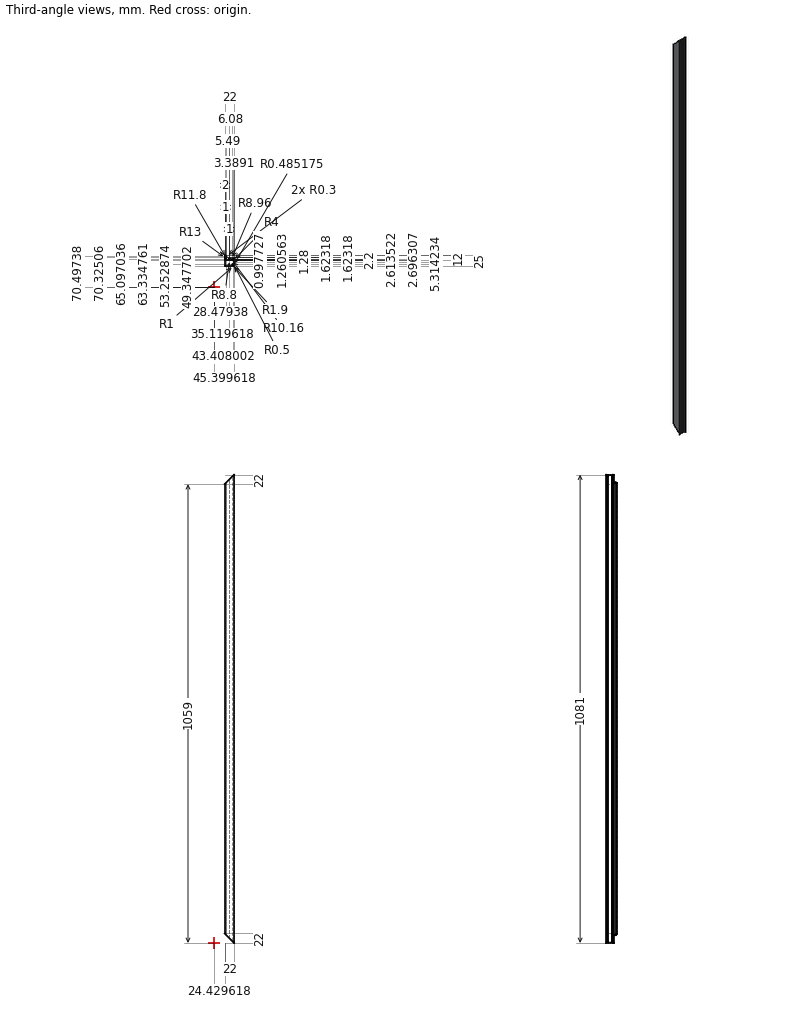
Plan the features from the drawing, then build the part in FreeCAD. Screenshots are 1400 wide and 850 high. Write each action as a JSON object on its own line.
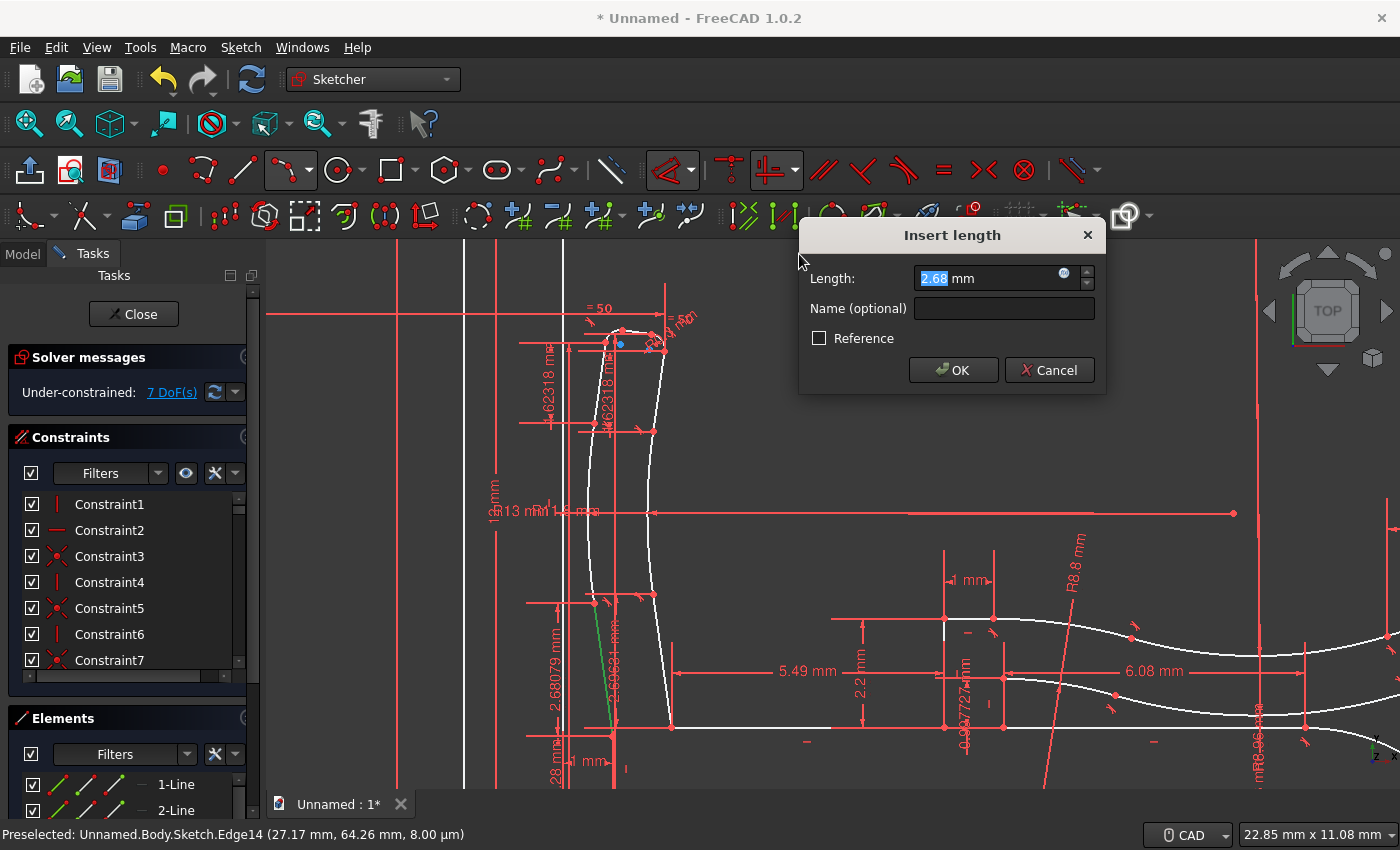
{"action": "type", "text": "2.613522"}
{"action": "key", "text": "Return"}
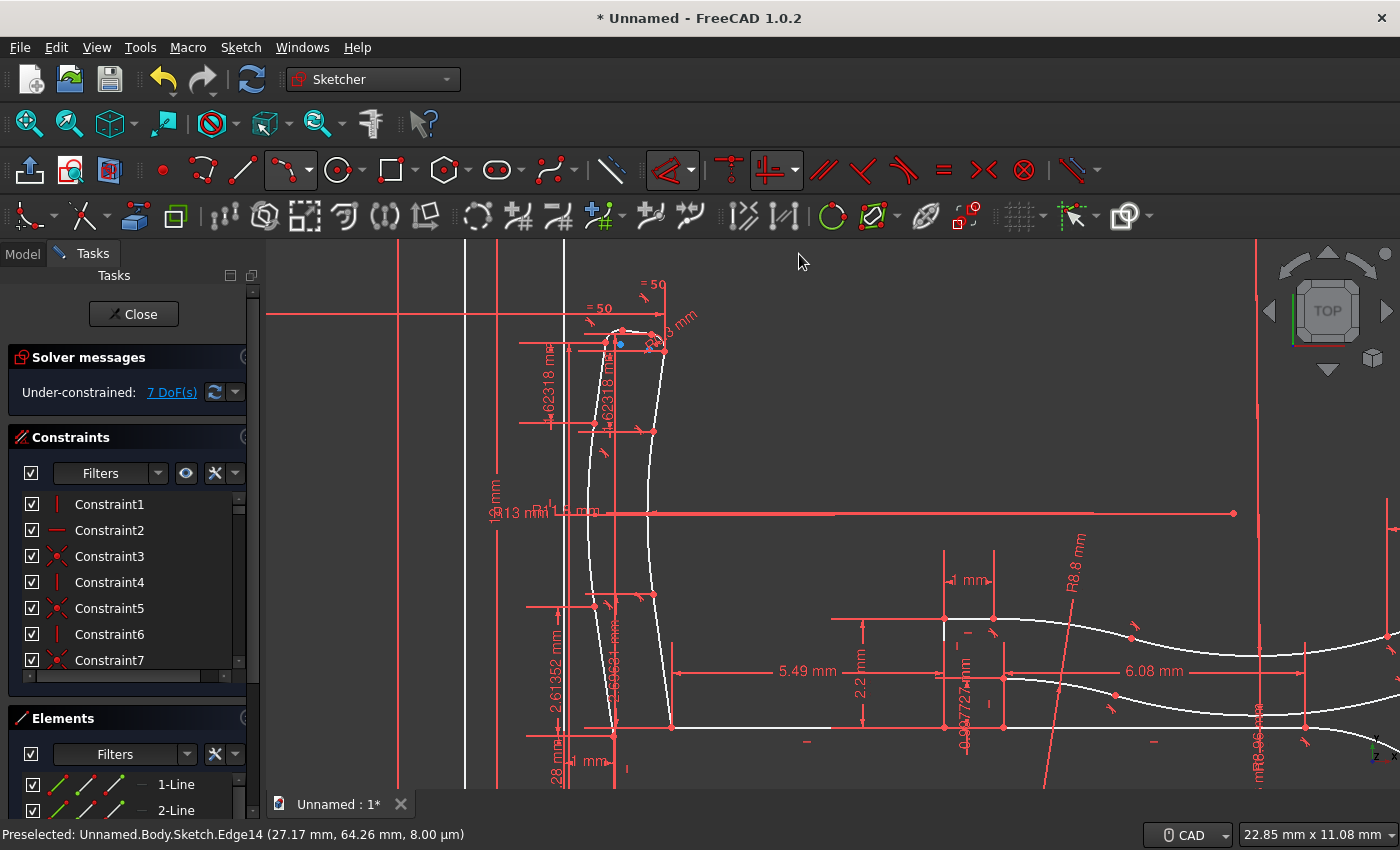
{"action": "scroll", "coordinate": [659, 382], "scroll_direction": "down", "scroll_amount": 6}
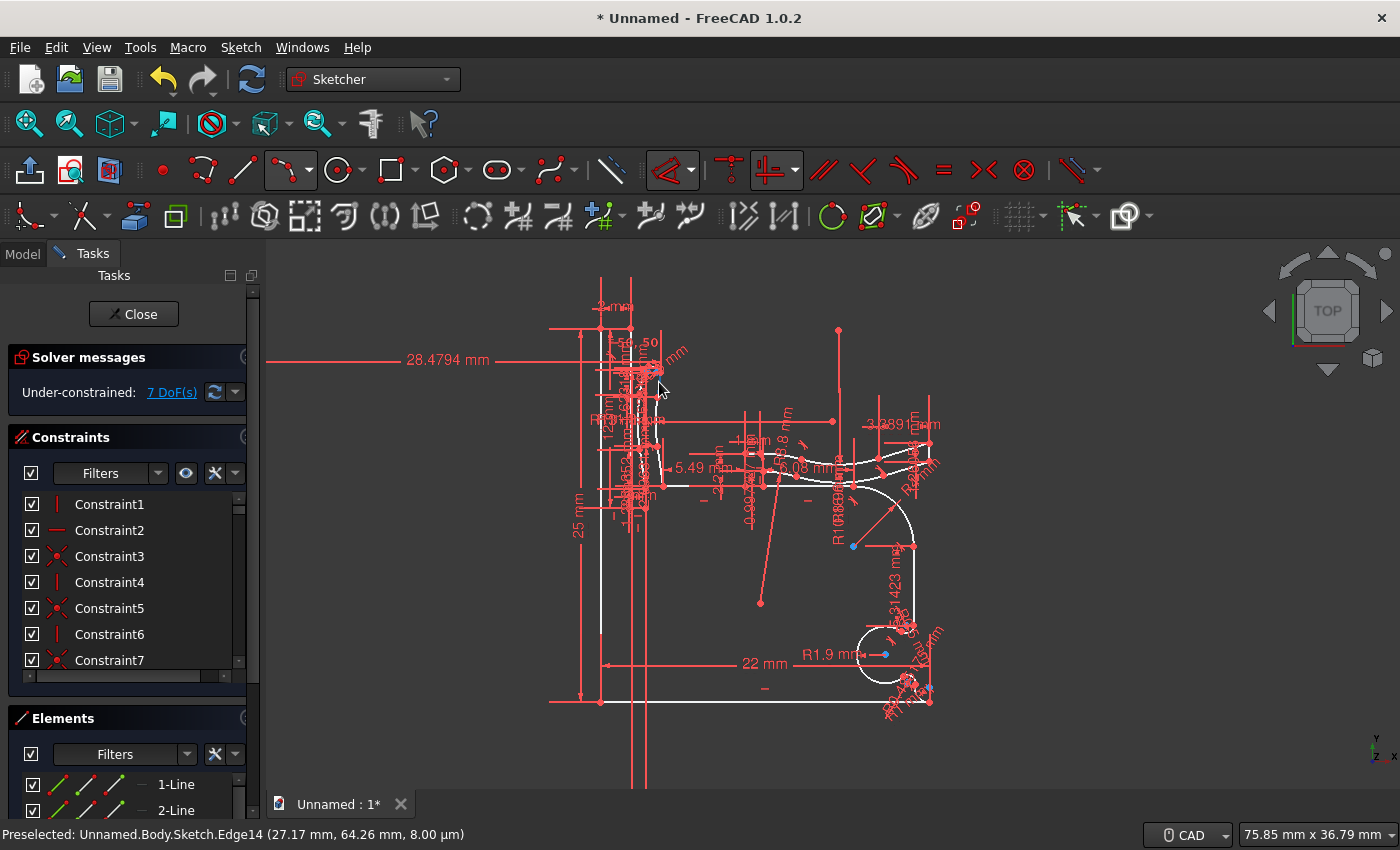
{"action": "scroll", "coordinate": [914, 626], "scroll_direction": "up", "scroll_amount": 3}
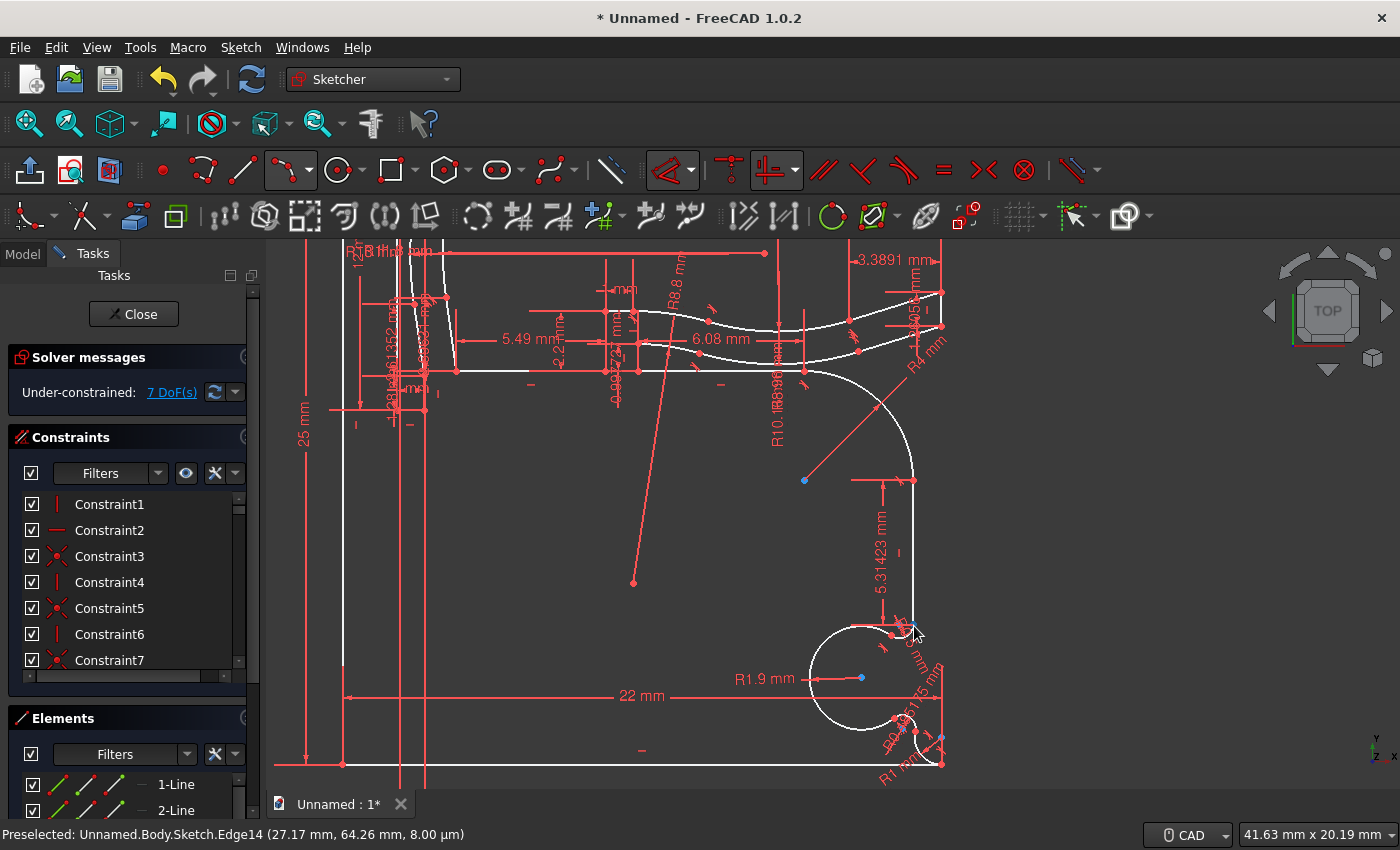
{"action": "left_click", "coordinate": [913, 625]}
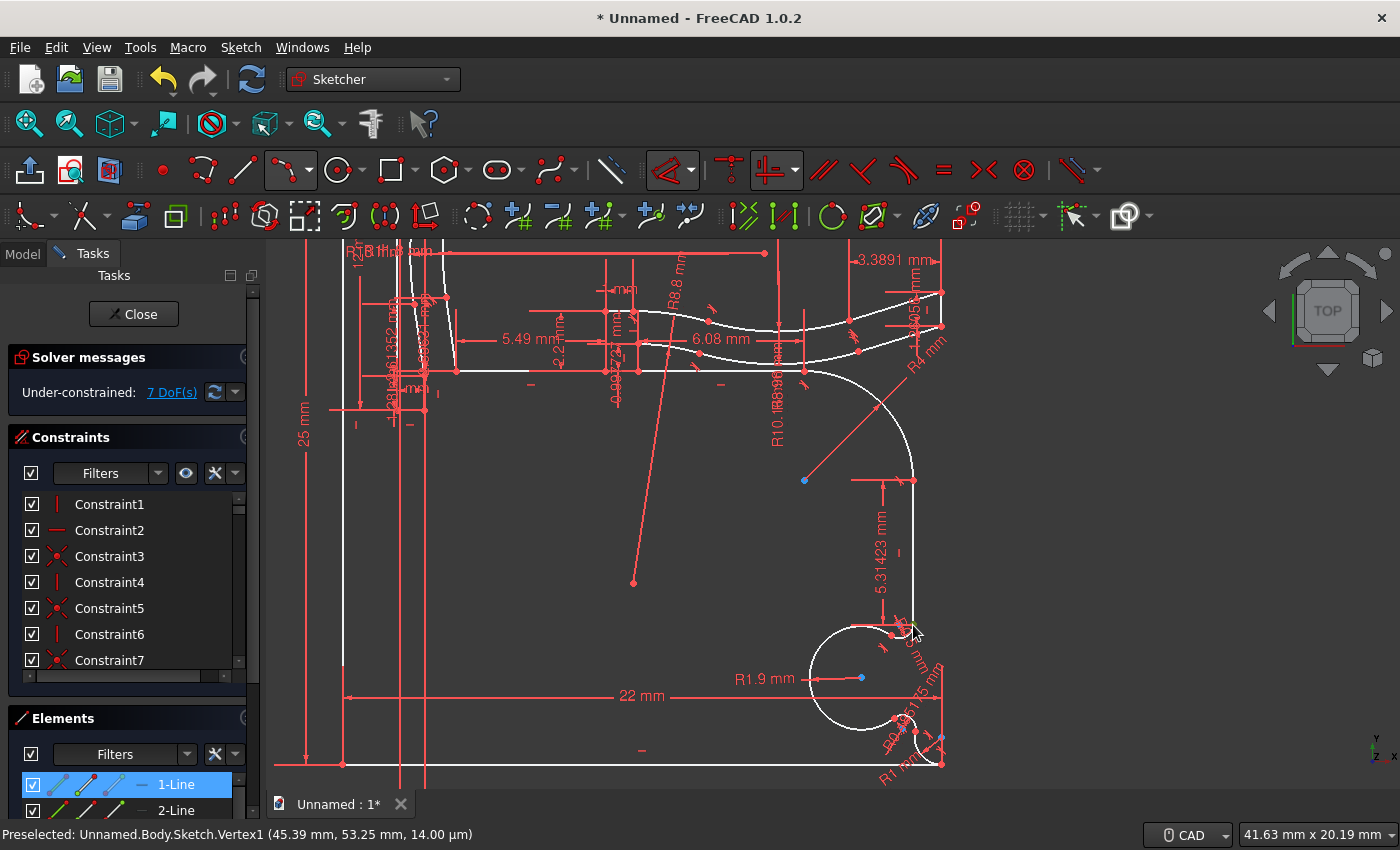
{"action": "left_click", "coordinate": [694, 170]}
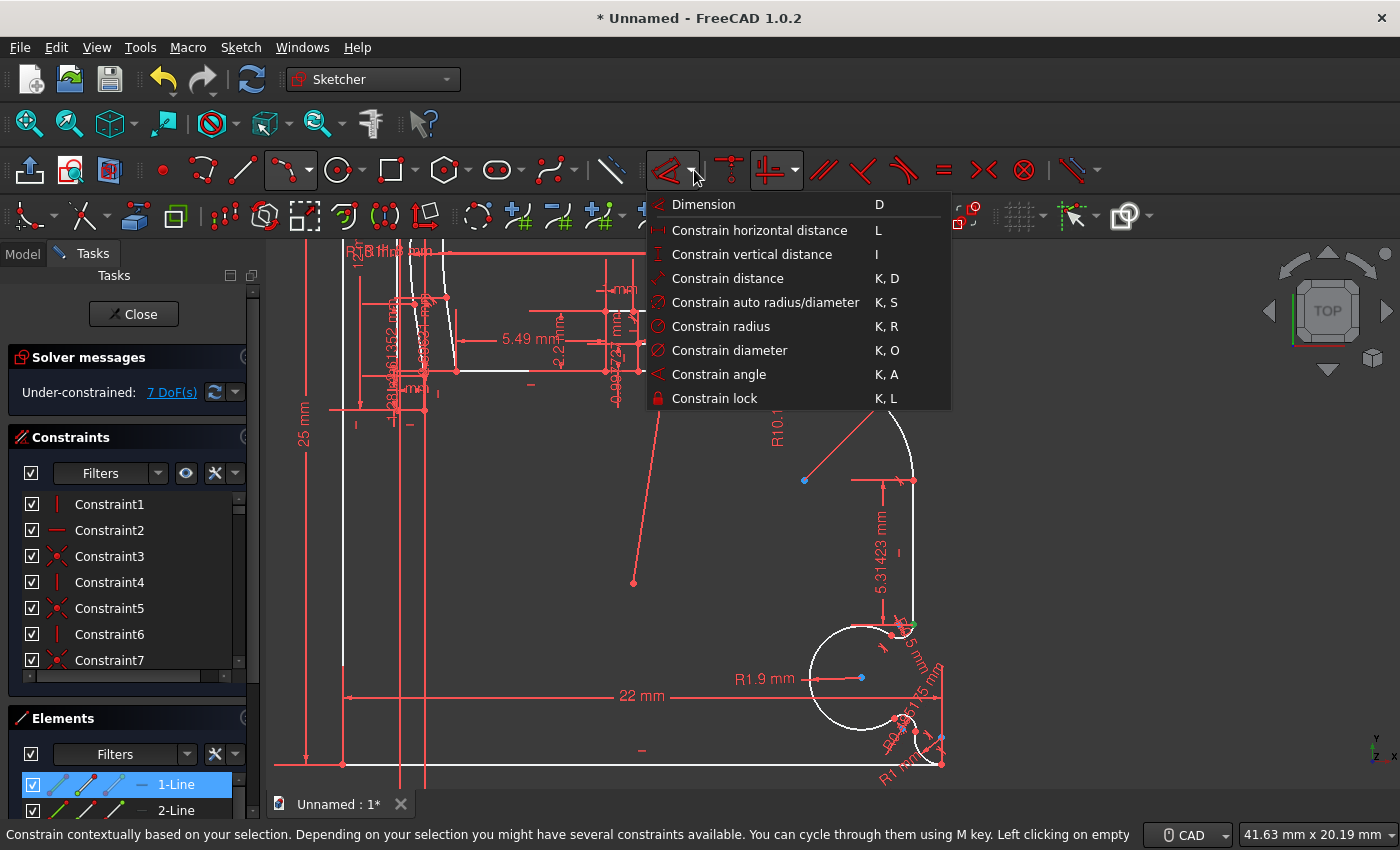
{"action": "left_click", "coordinate": [799, 230]}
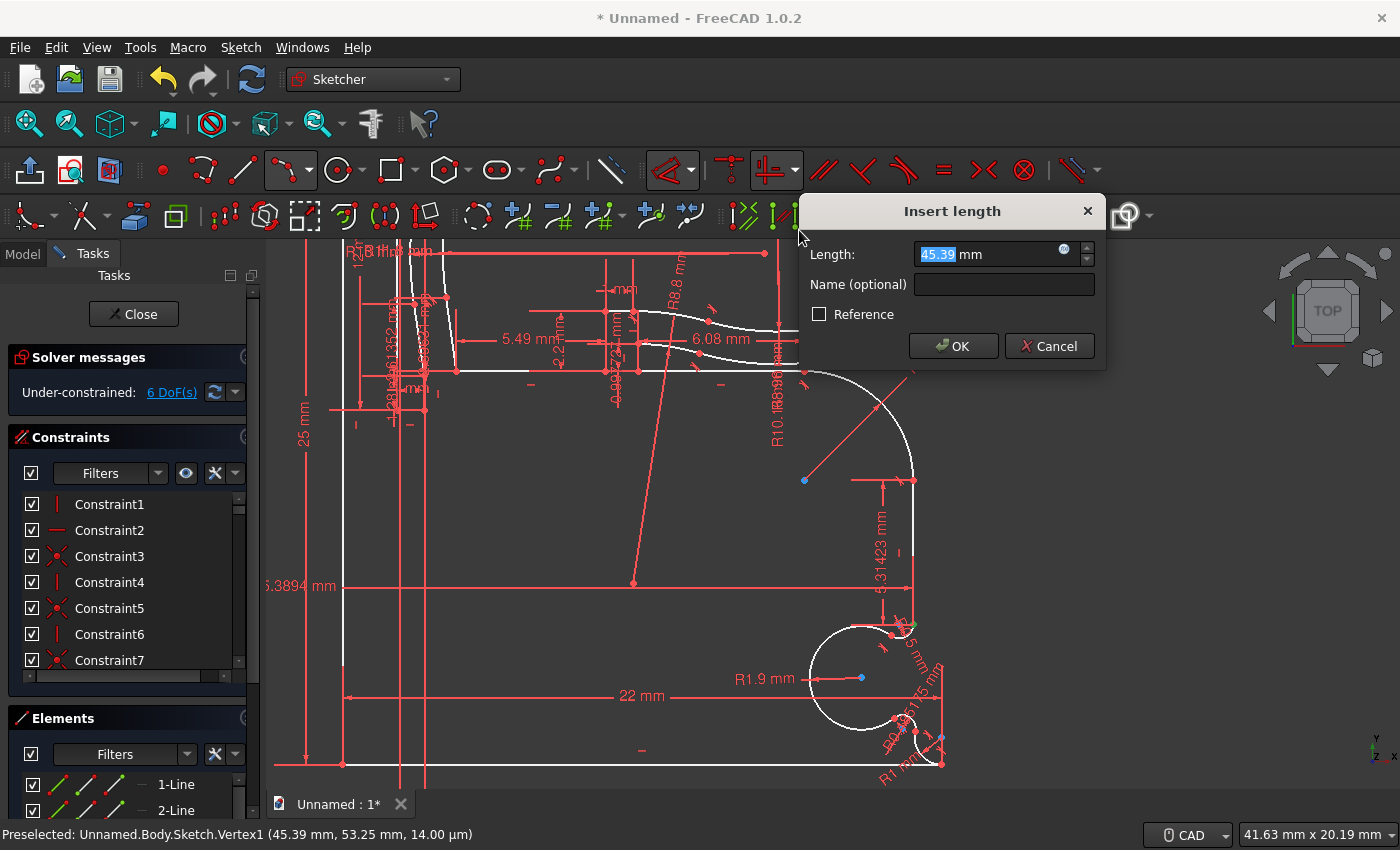
{"action": "type", "text": "45.399618"}
{"action": "key", "text": "Return"}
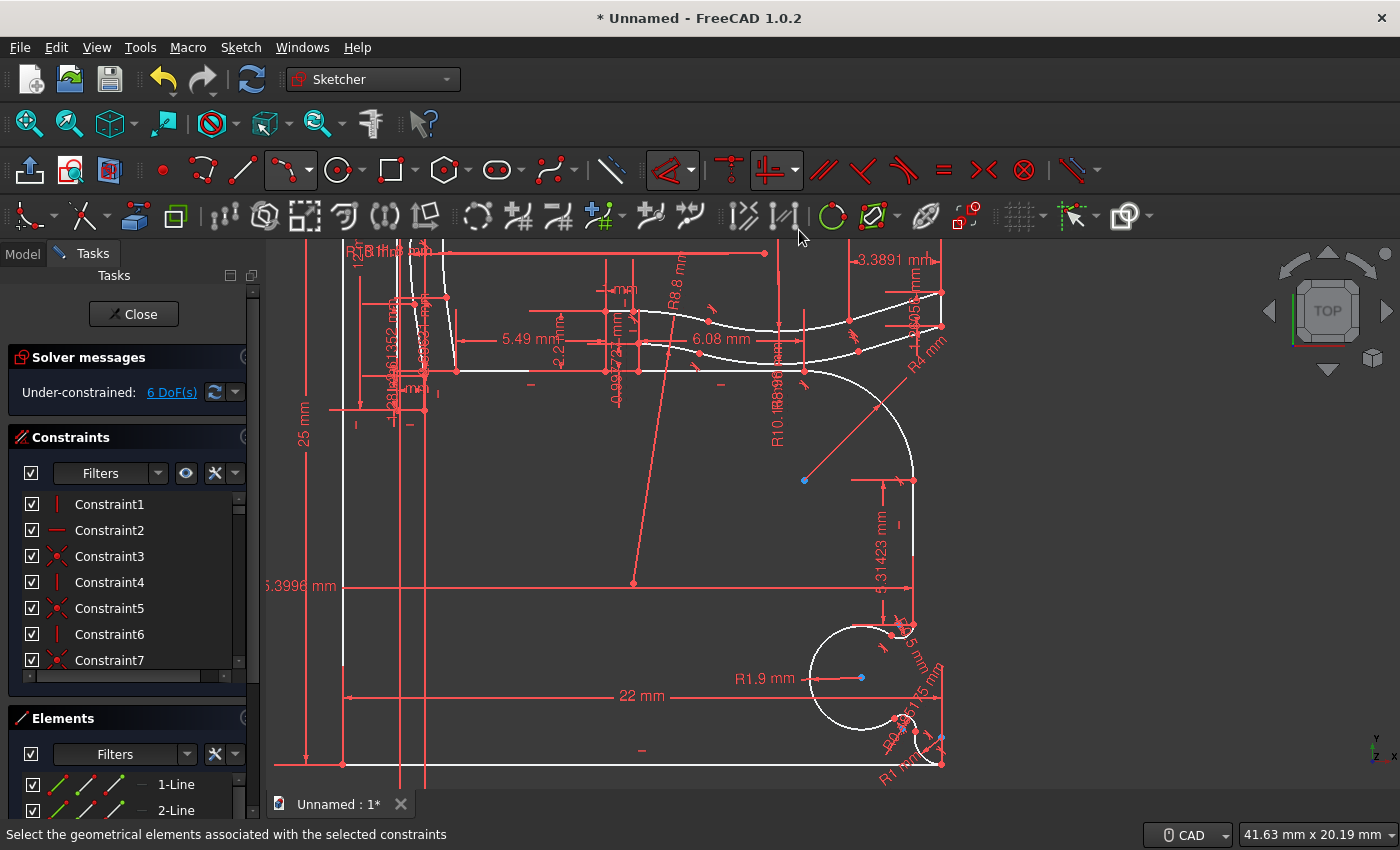
{"action": "left_click", "coordinate": [913, 625]}